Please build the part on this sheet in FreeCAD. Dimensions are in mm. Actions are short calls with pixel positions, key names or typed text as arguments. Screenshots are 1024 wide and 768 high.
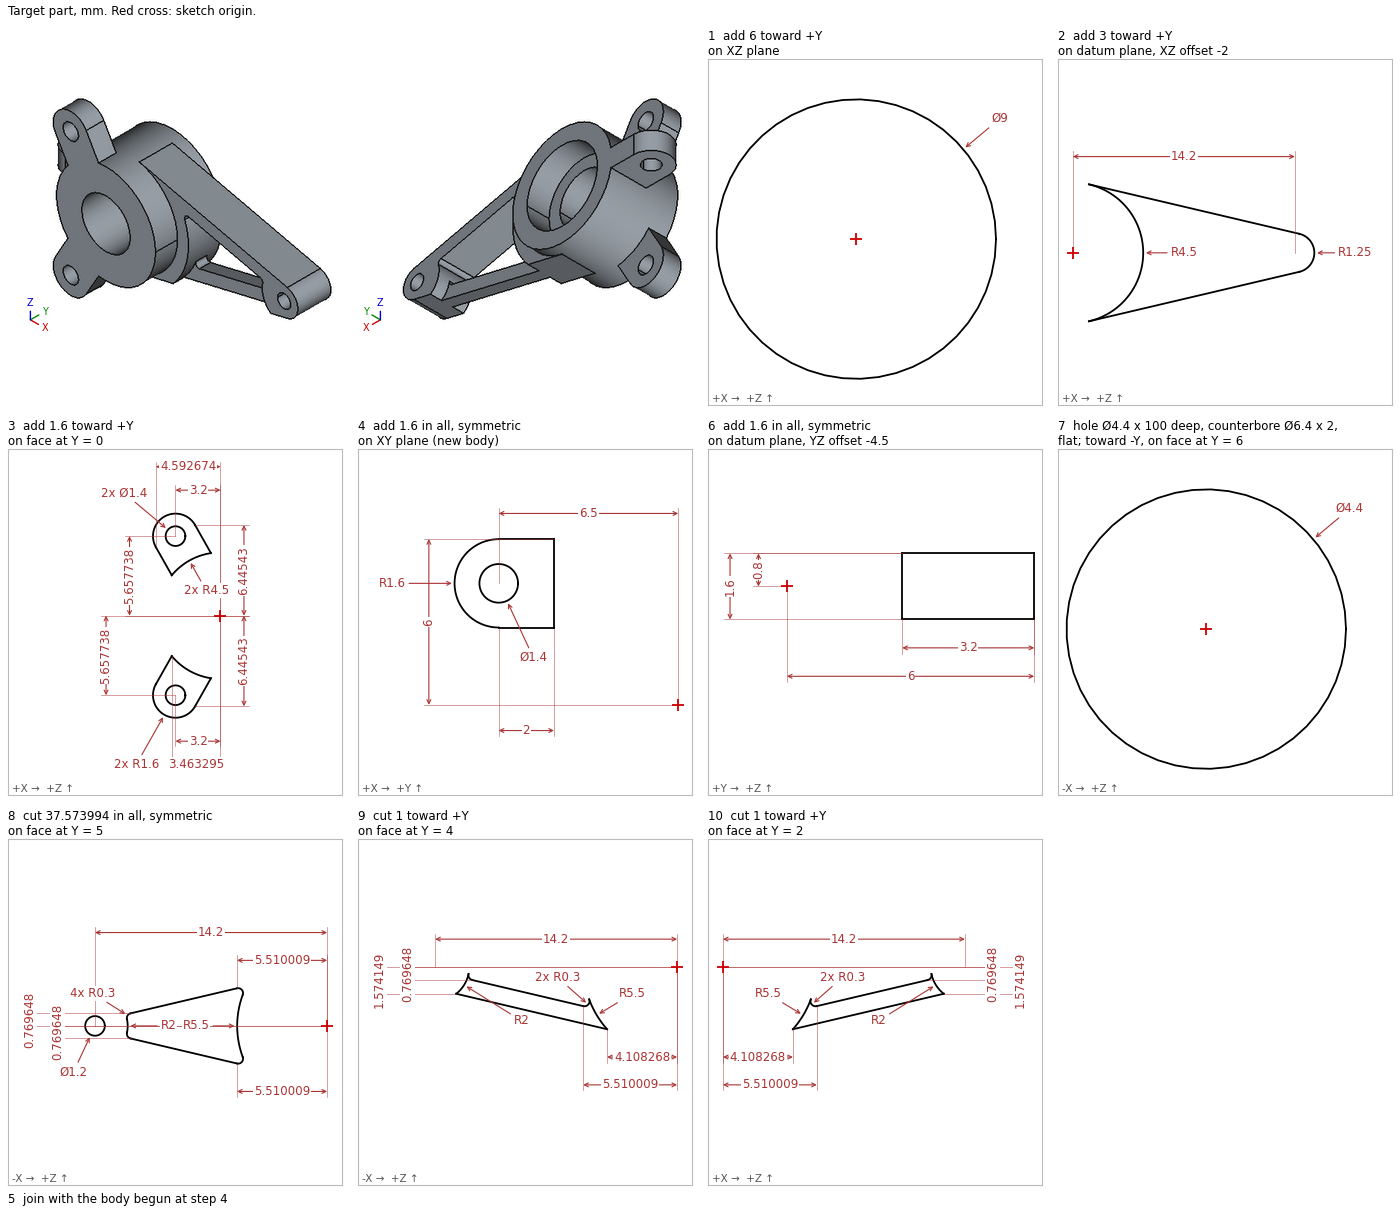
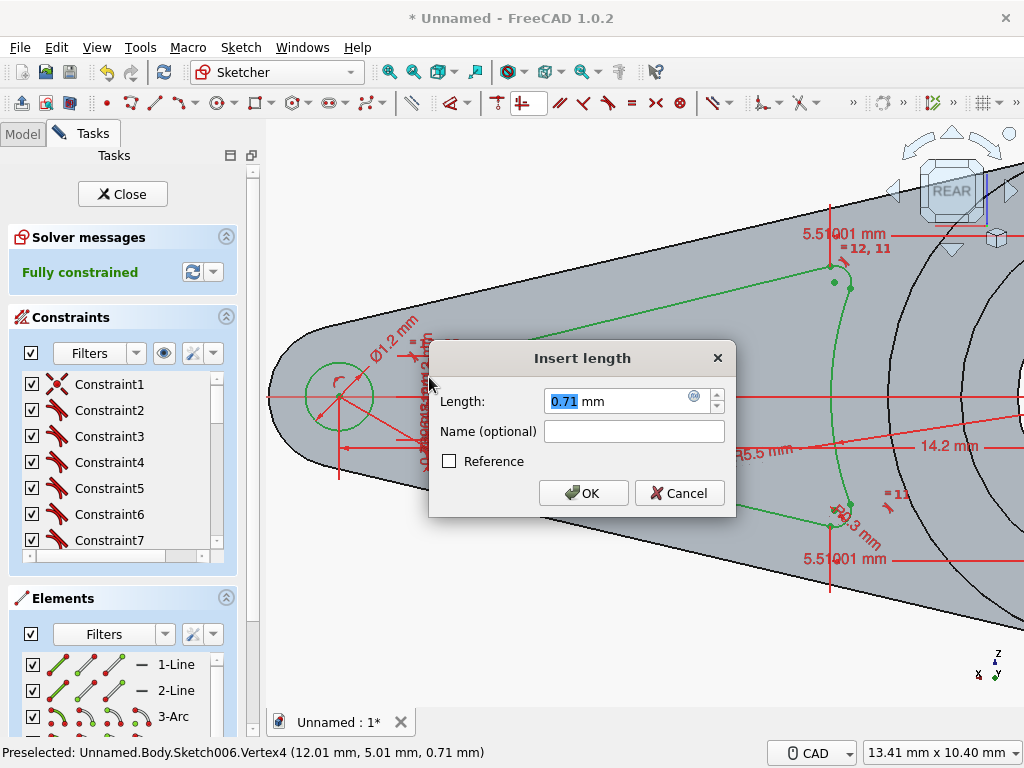
text(0.769648)
key(Return)
key(Escape)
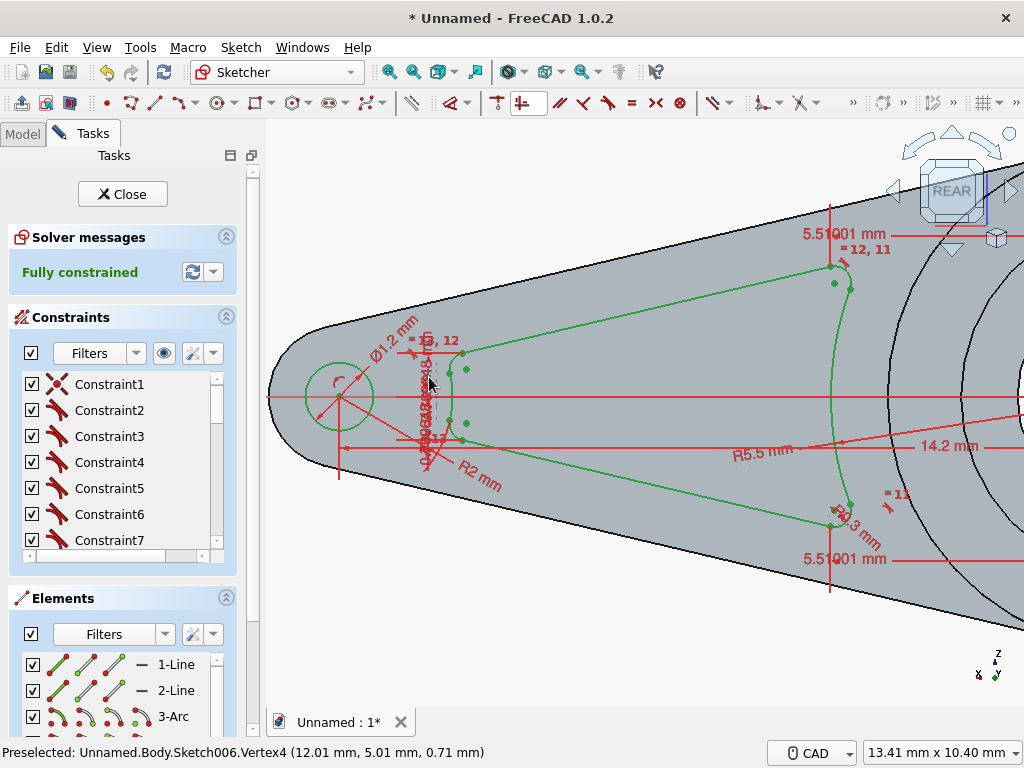
click(123, 194)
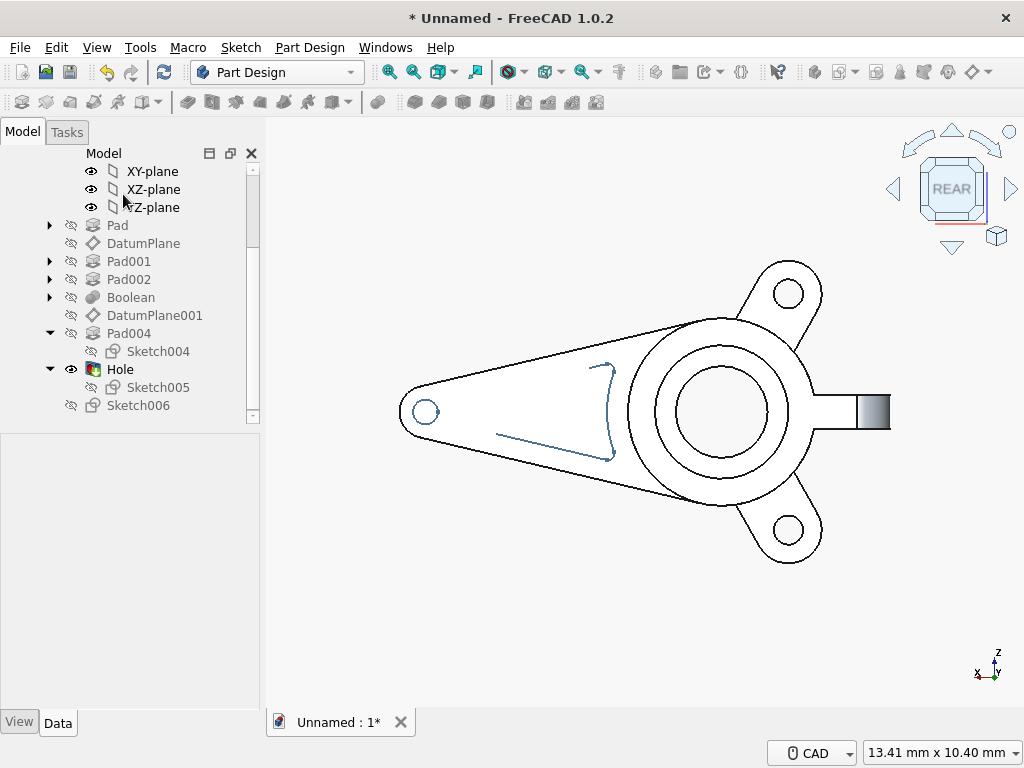
click(188, 102)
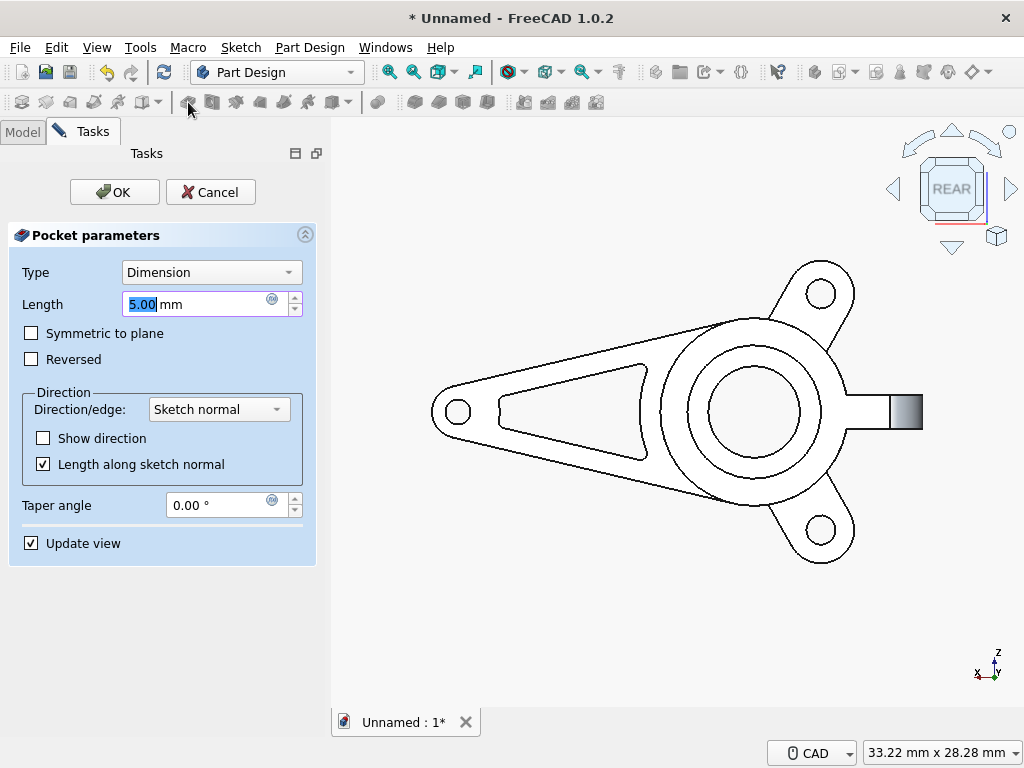
text(37.573994)
key(Tab)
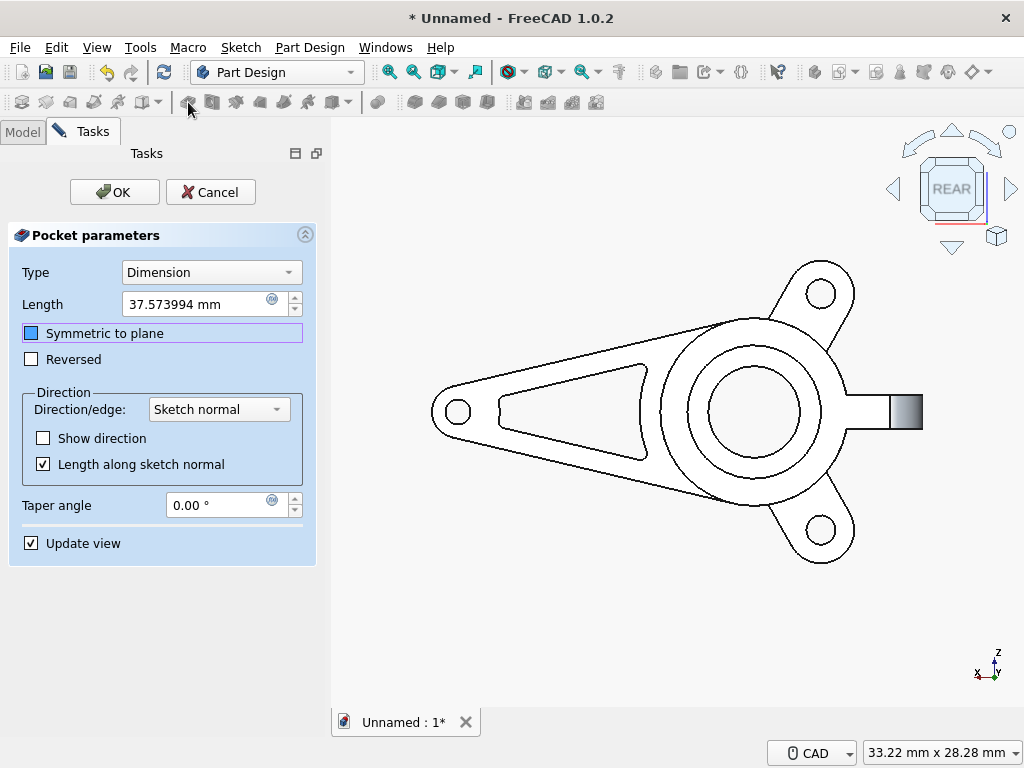
click(30, 333)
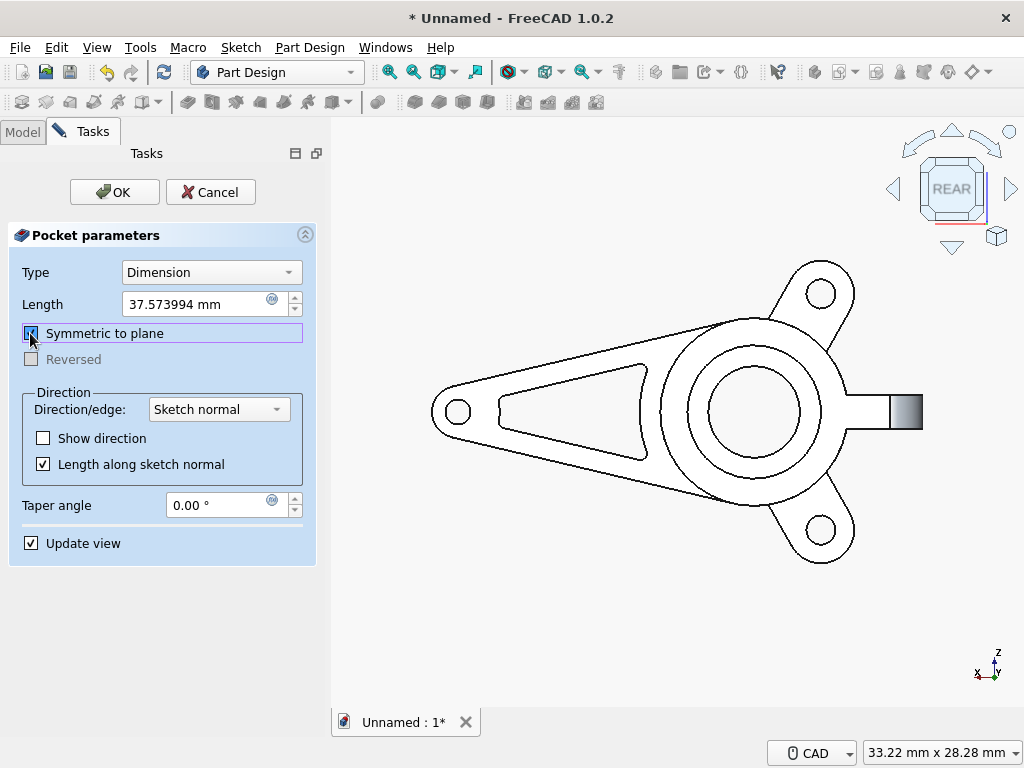
click(115, 192)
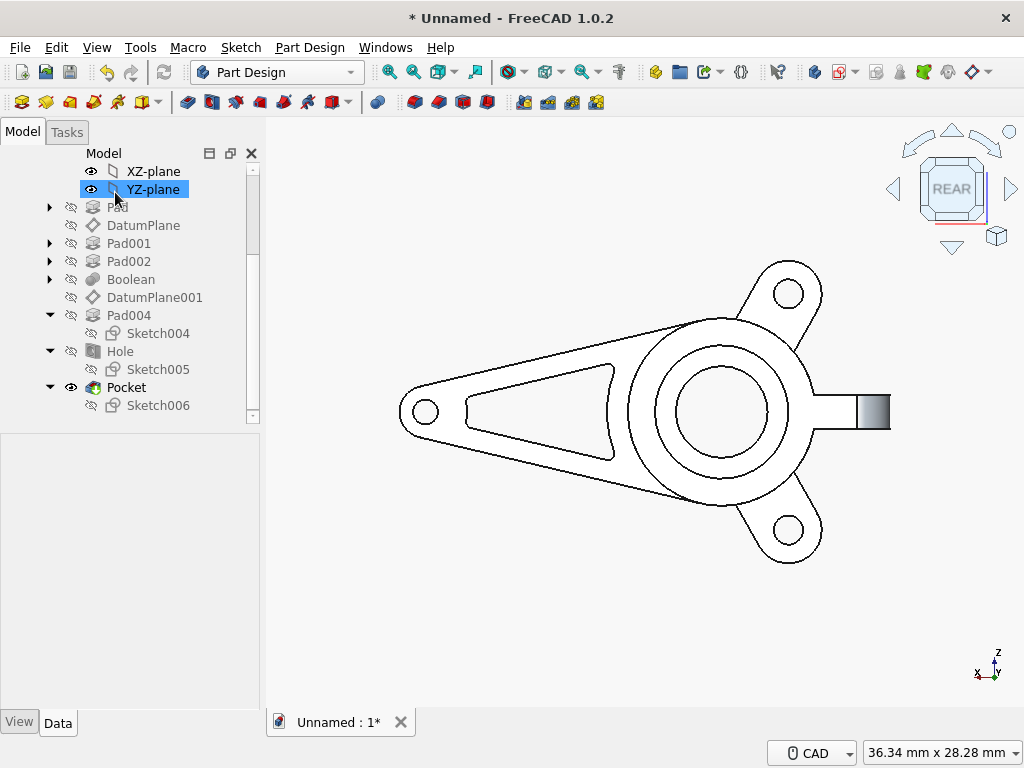
click(664, 411)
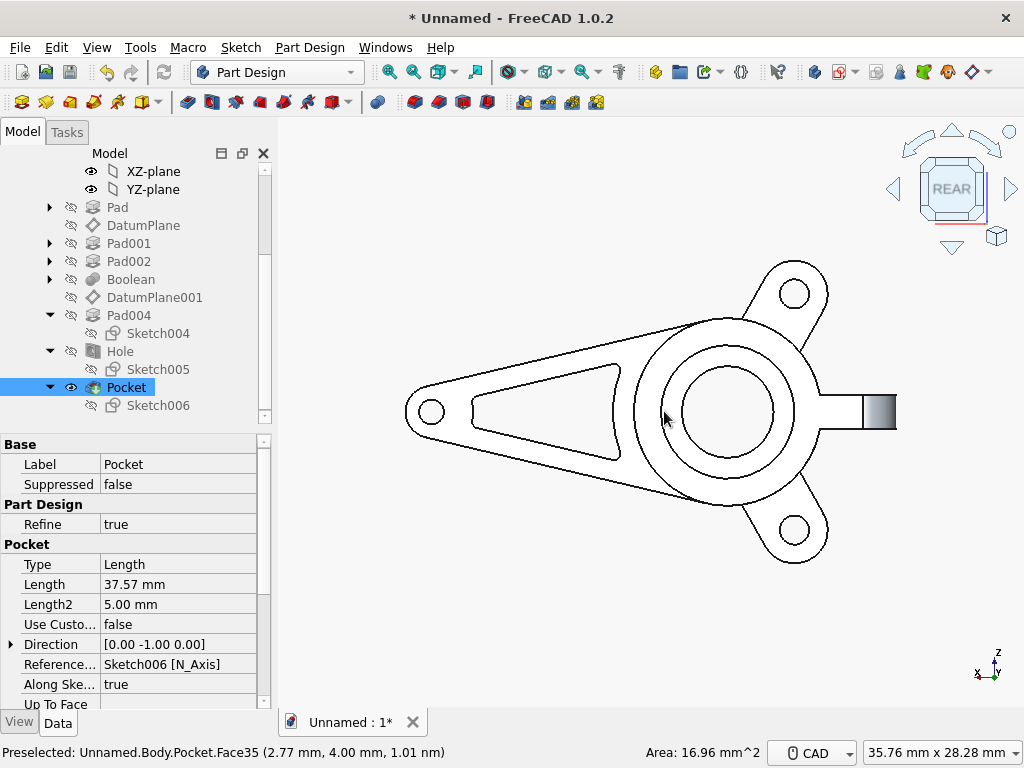
click(840, 72)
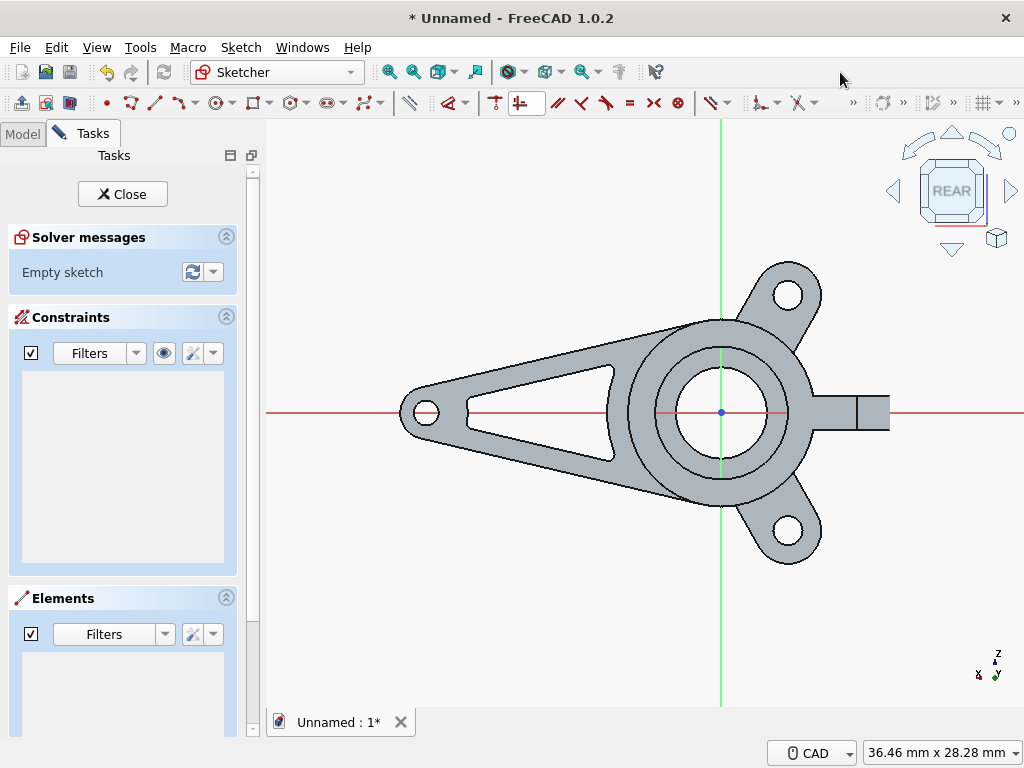
click(70, 104)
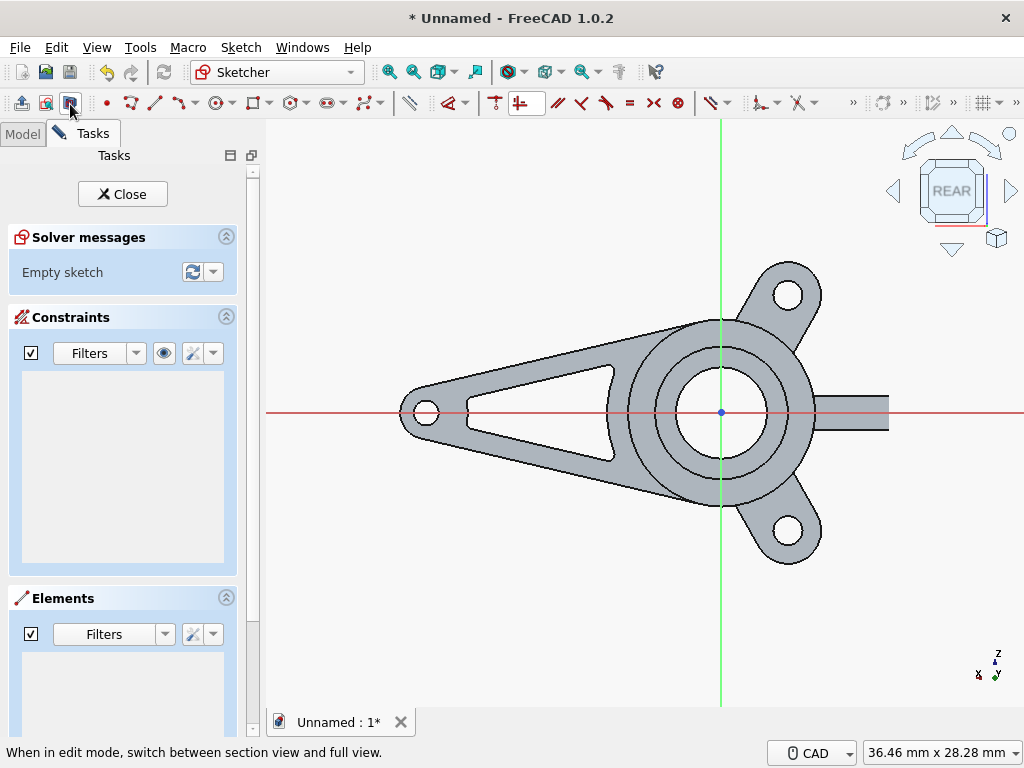
scroll(607, 528, up, 2)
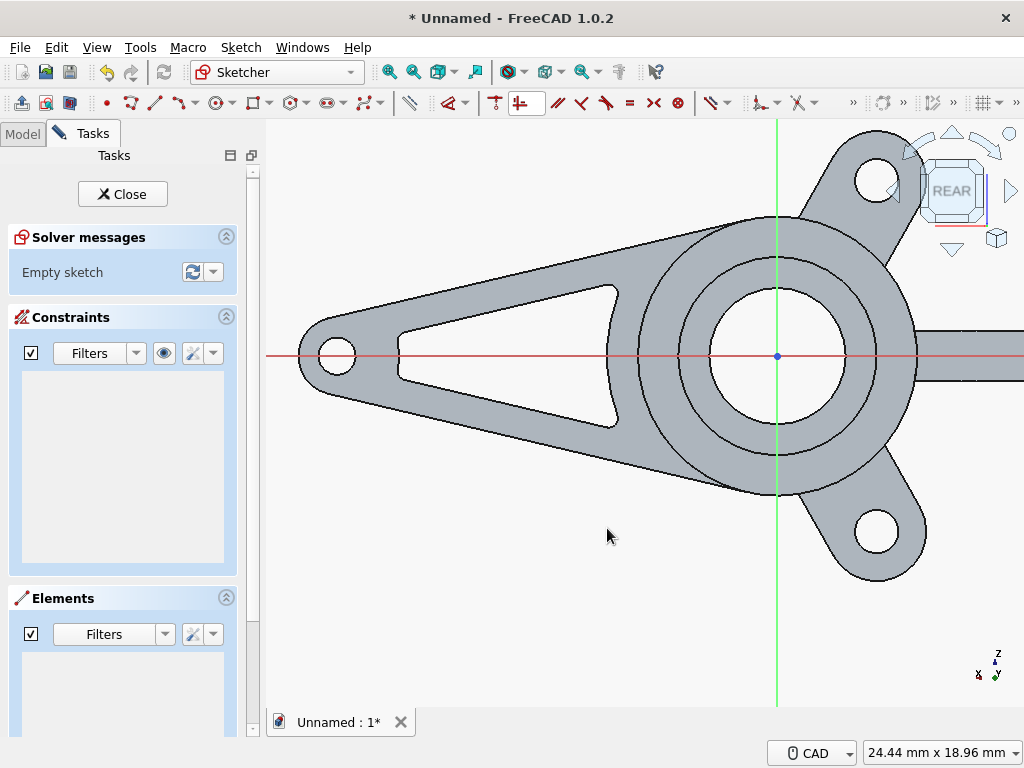
key(g)
key(l)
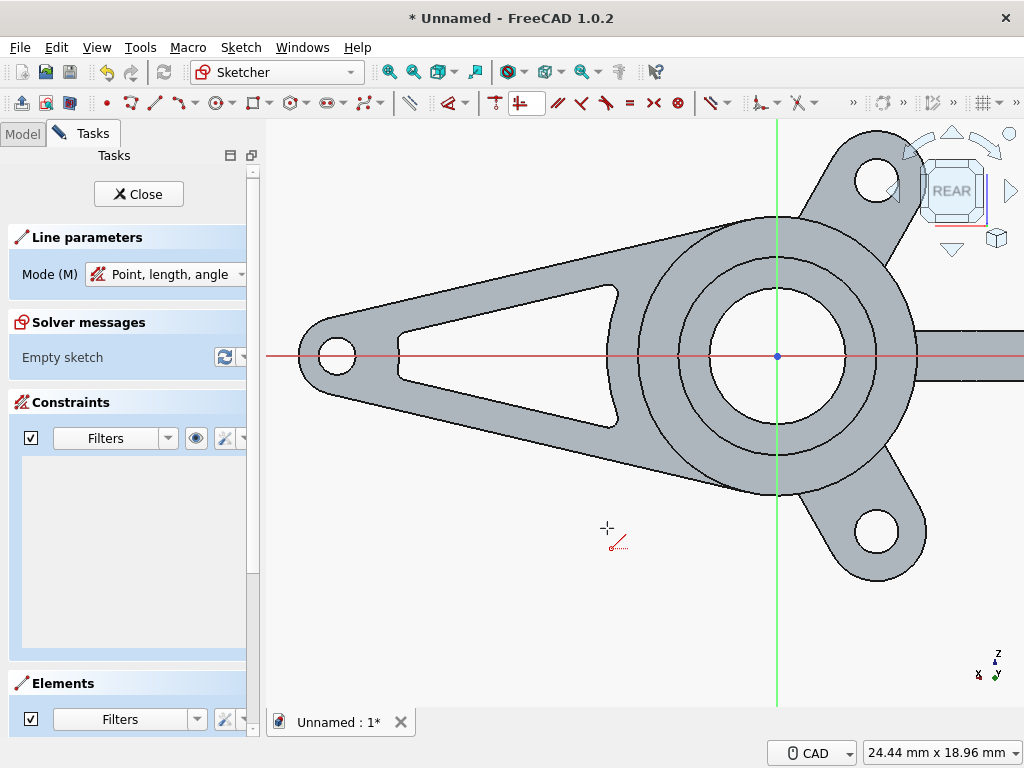
click(375, 405)
click(650, 470)